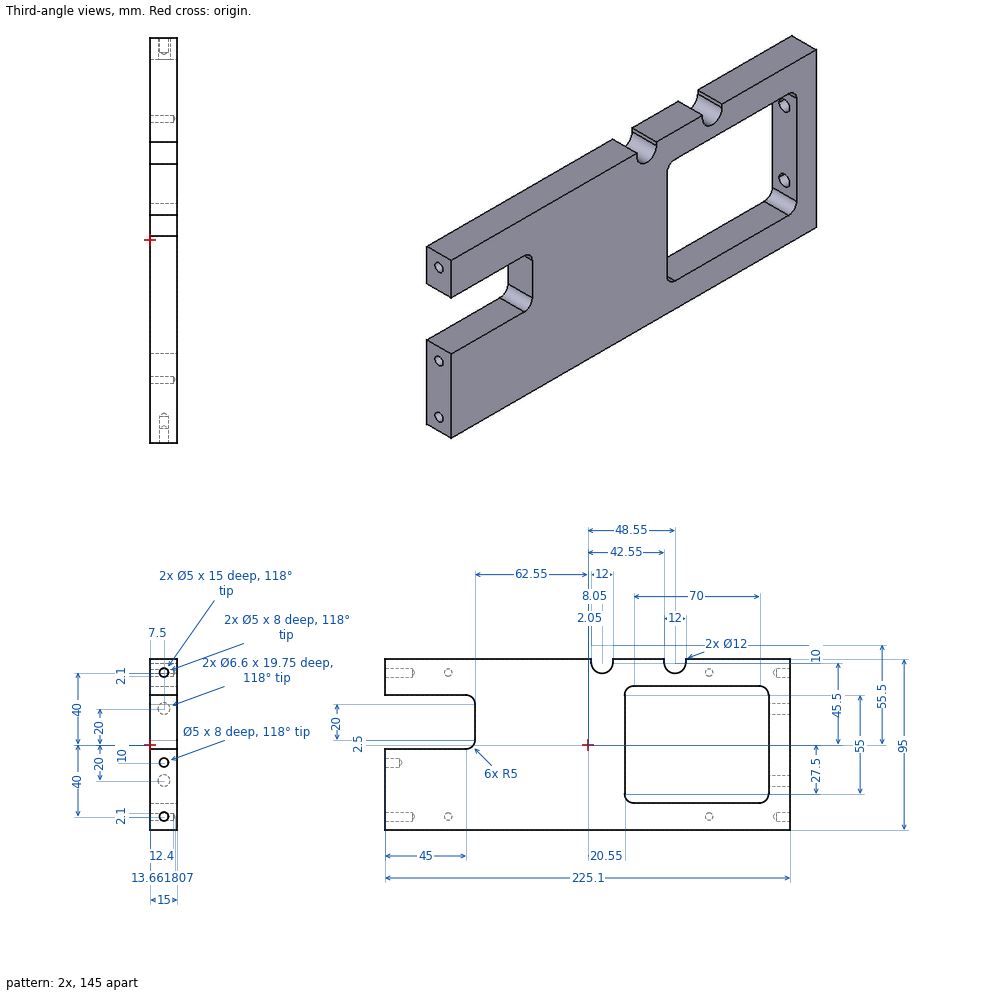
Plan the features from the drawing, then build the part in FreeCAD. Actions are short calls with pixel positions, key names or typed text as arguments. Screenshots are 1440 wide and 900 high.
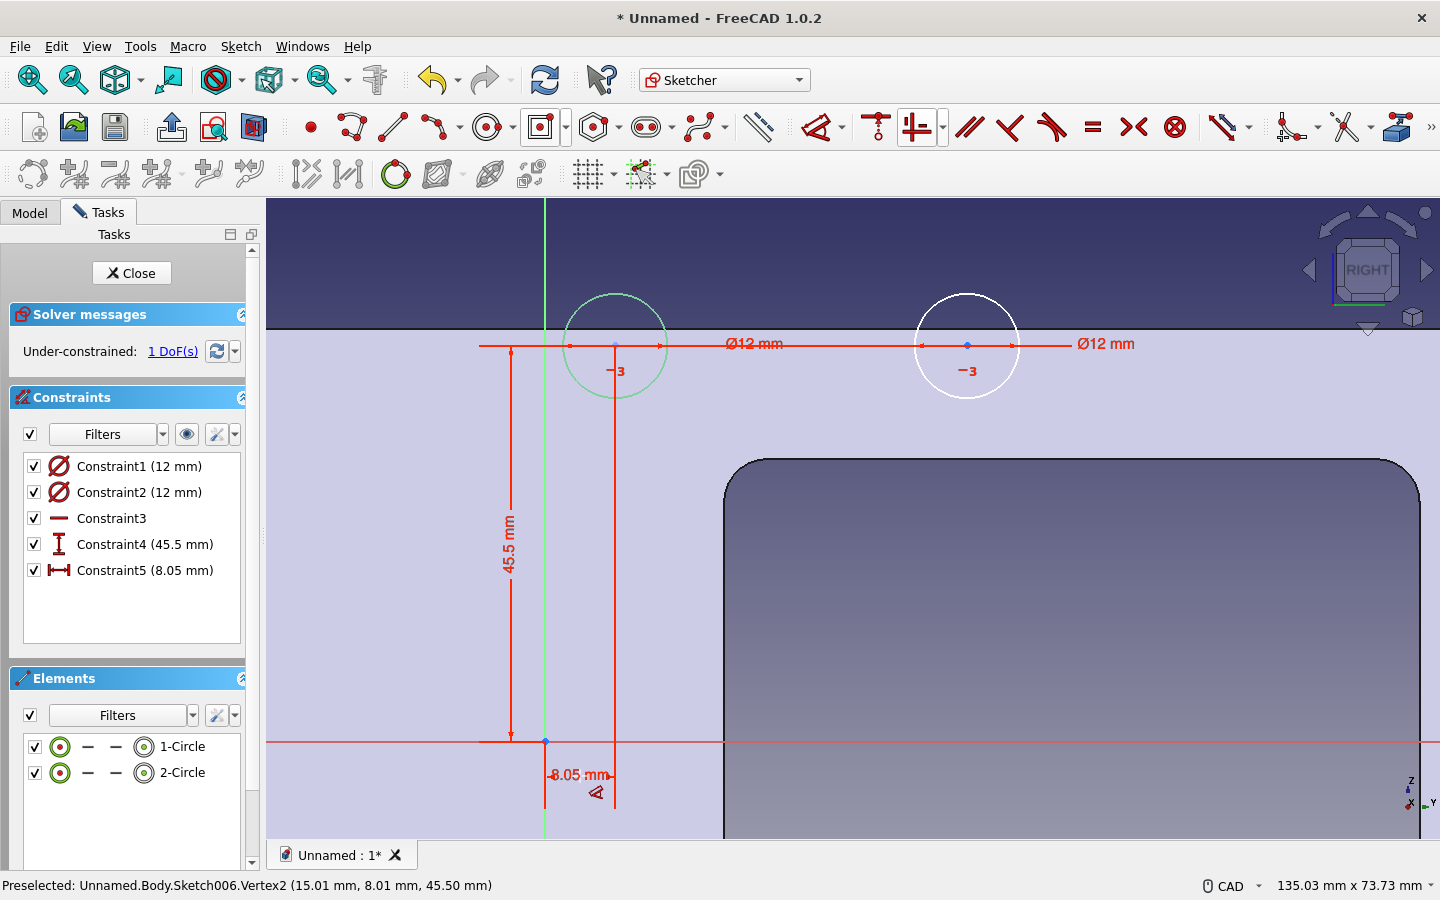
click(967, 346)
click(756, 776)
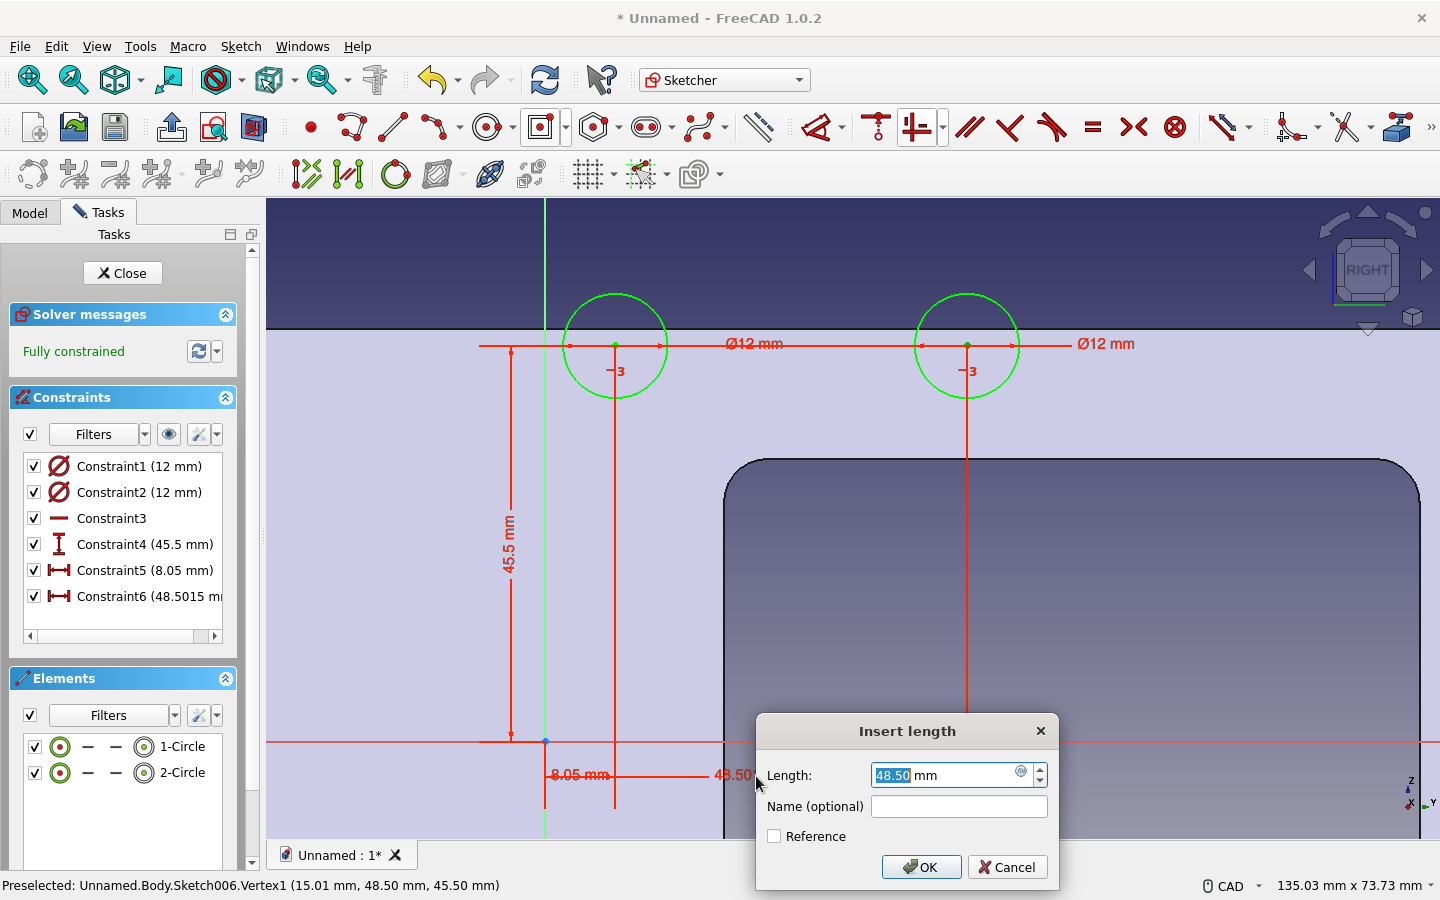
text(48.55)
key(Return)
key(Escape)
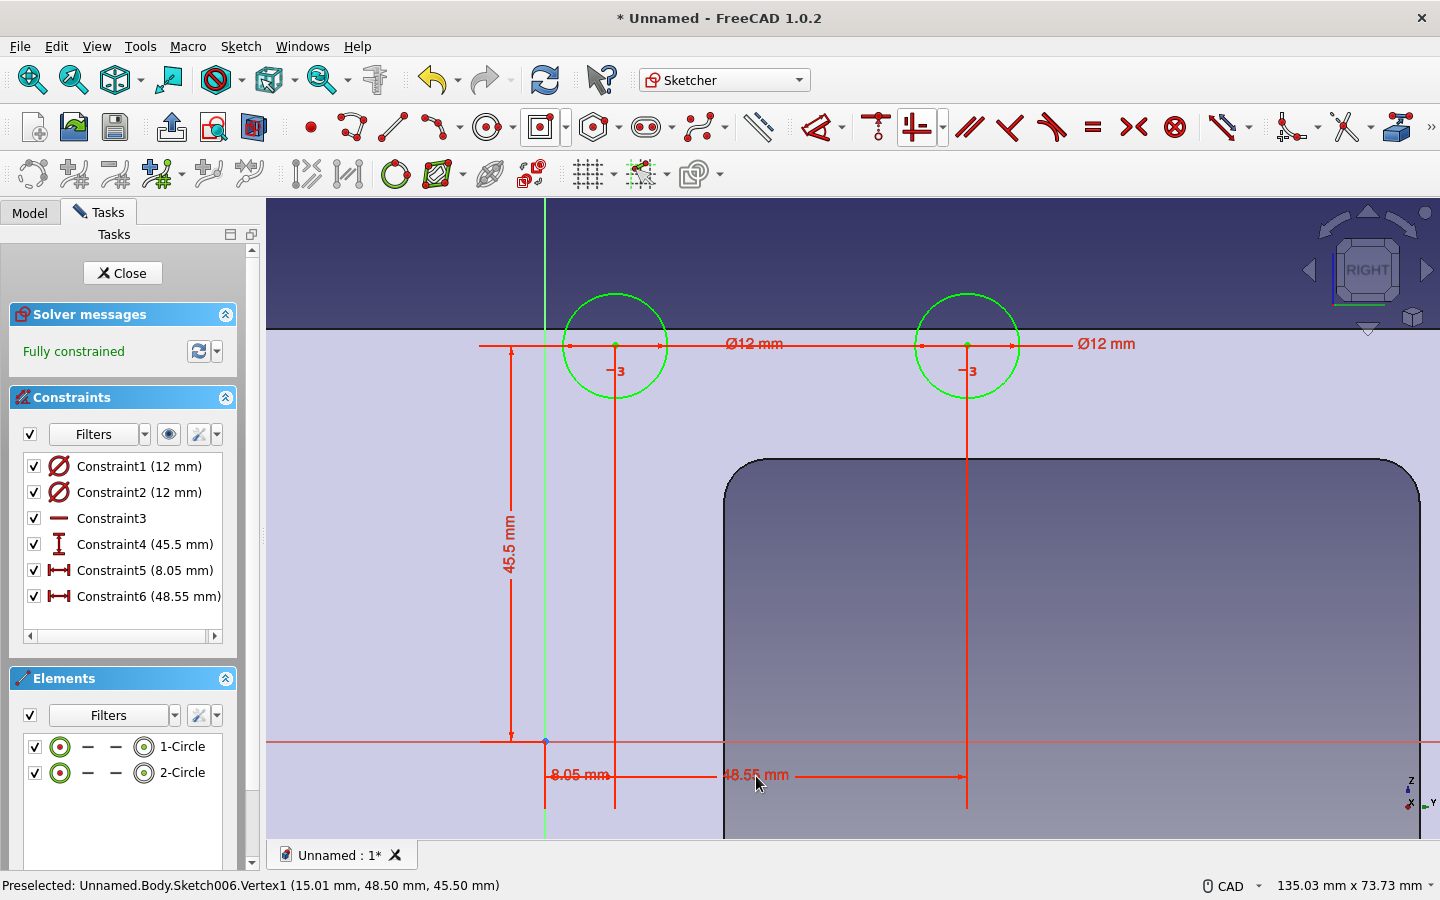
click(123, 273)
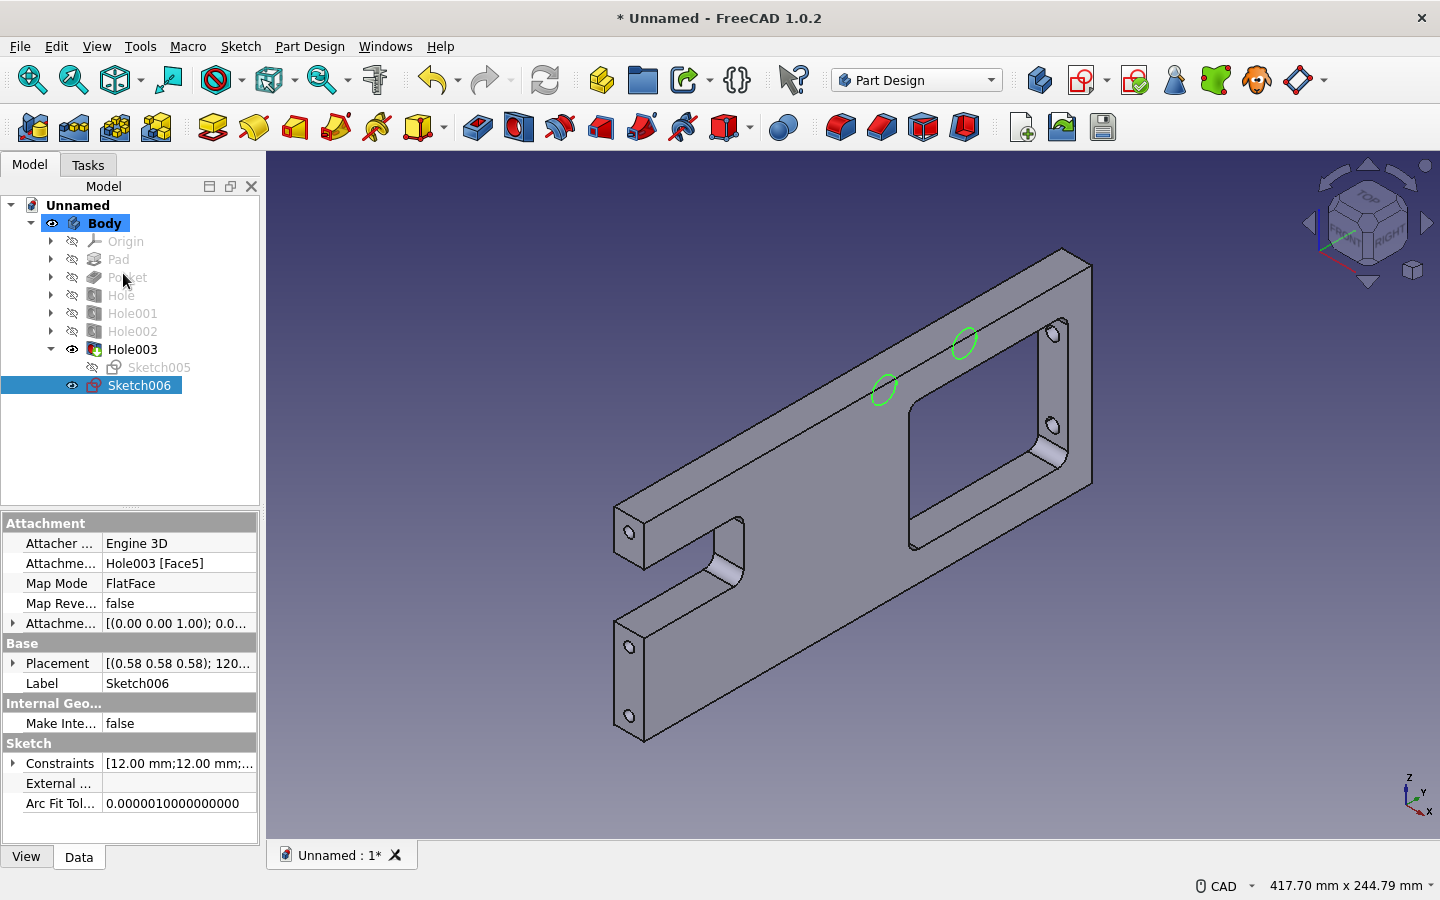
click(478, 128)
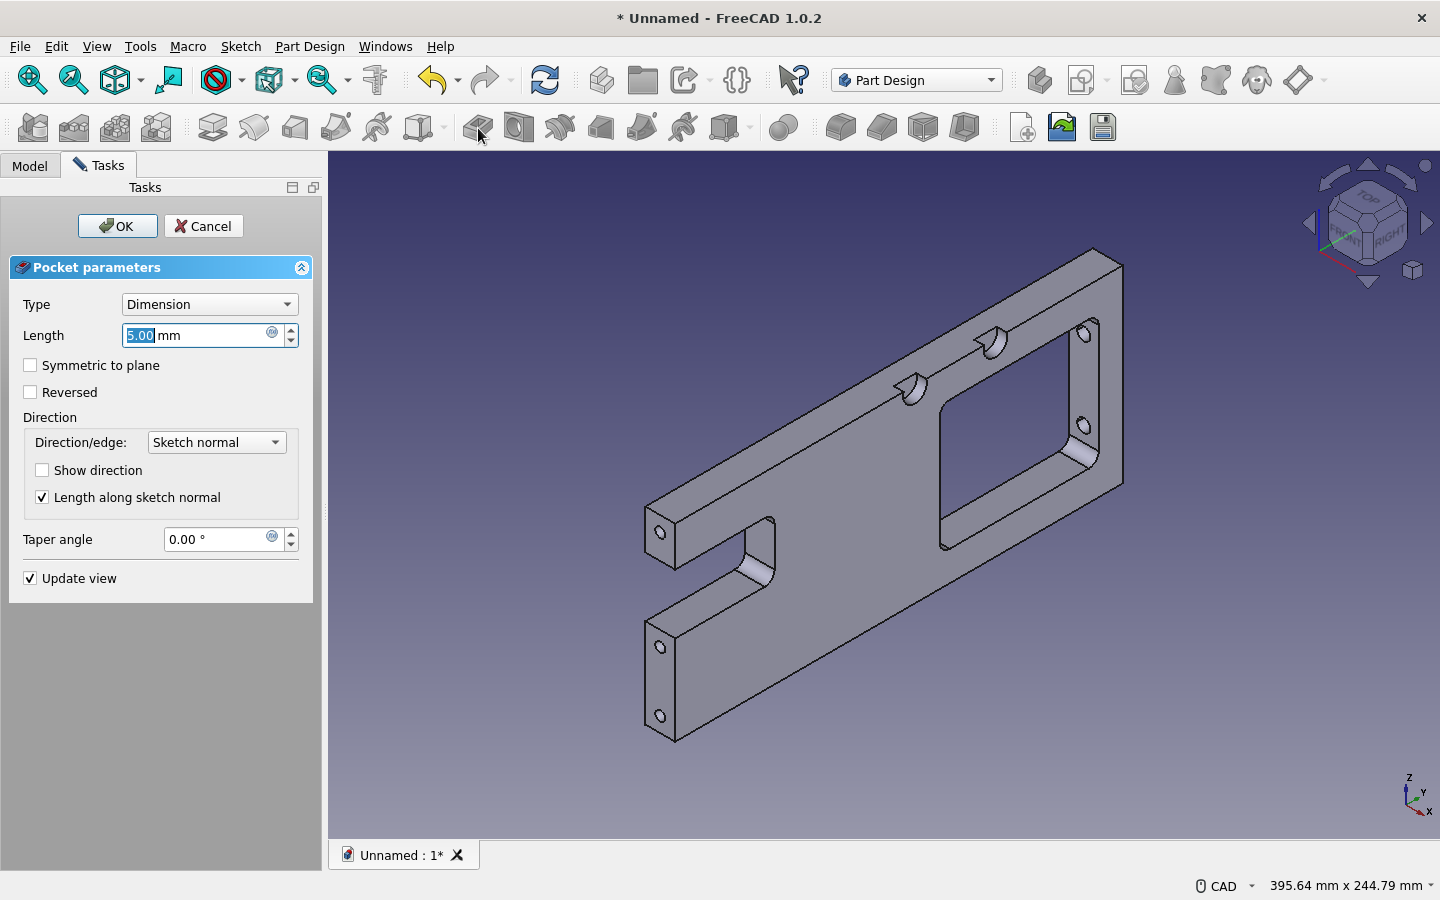
click(210, 304)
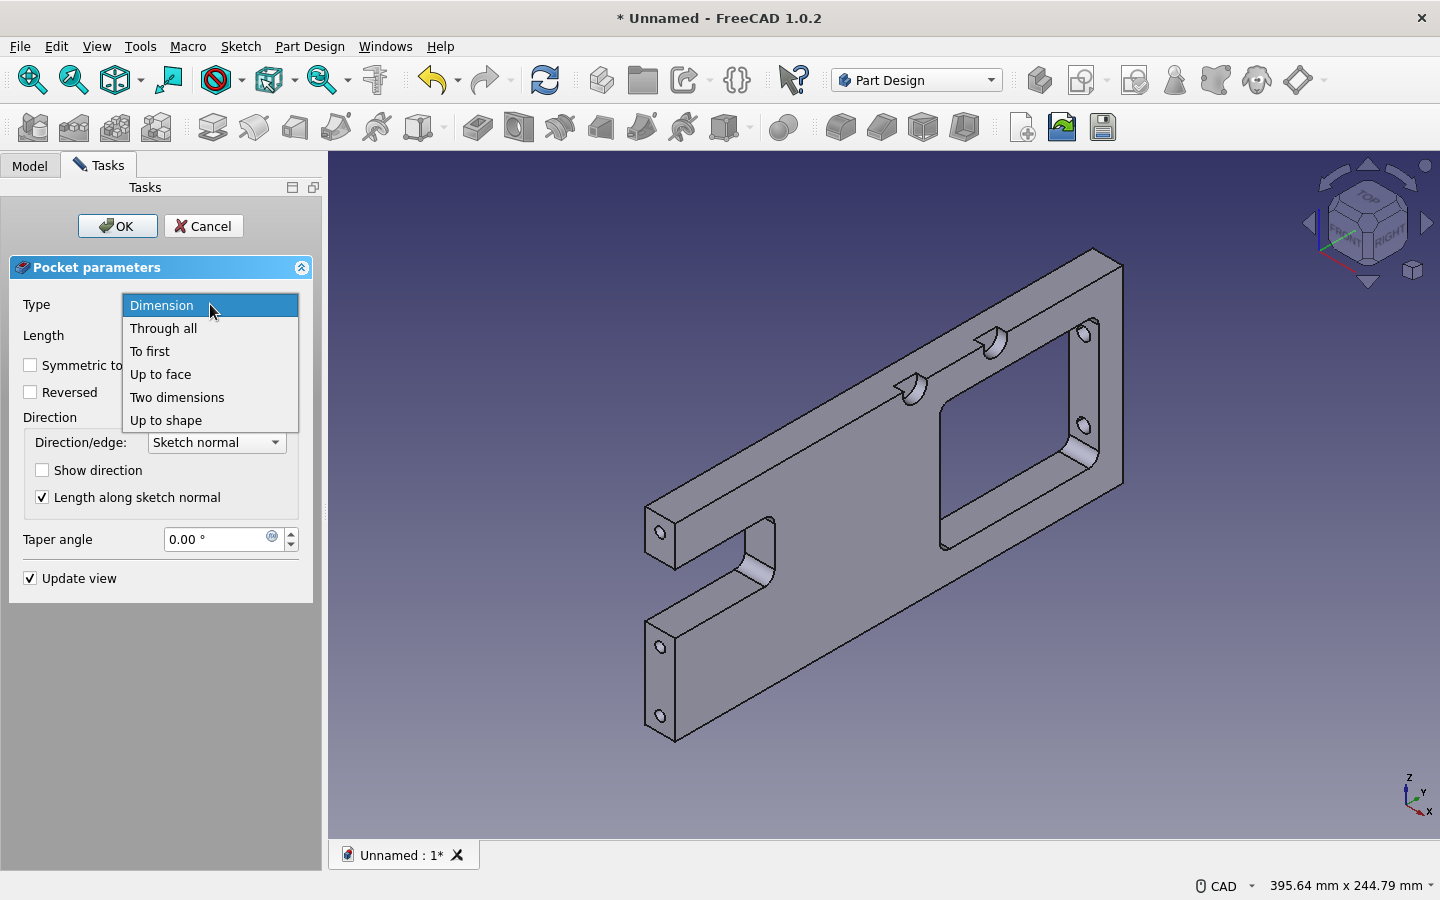
click(208, 328)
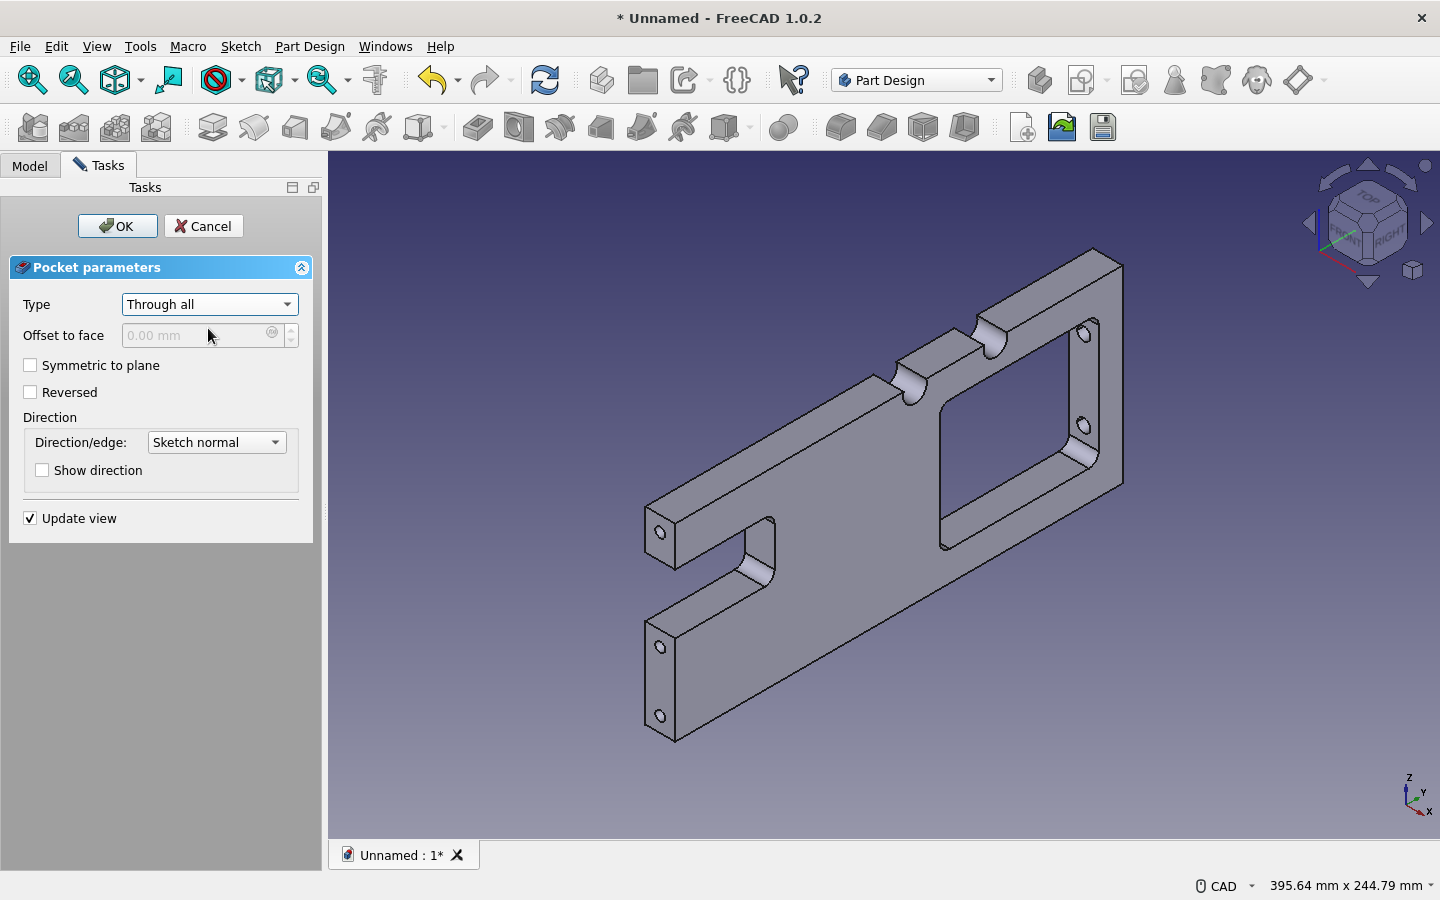
click(118, 226)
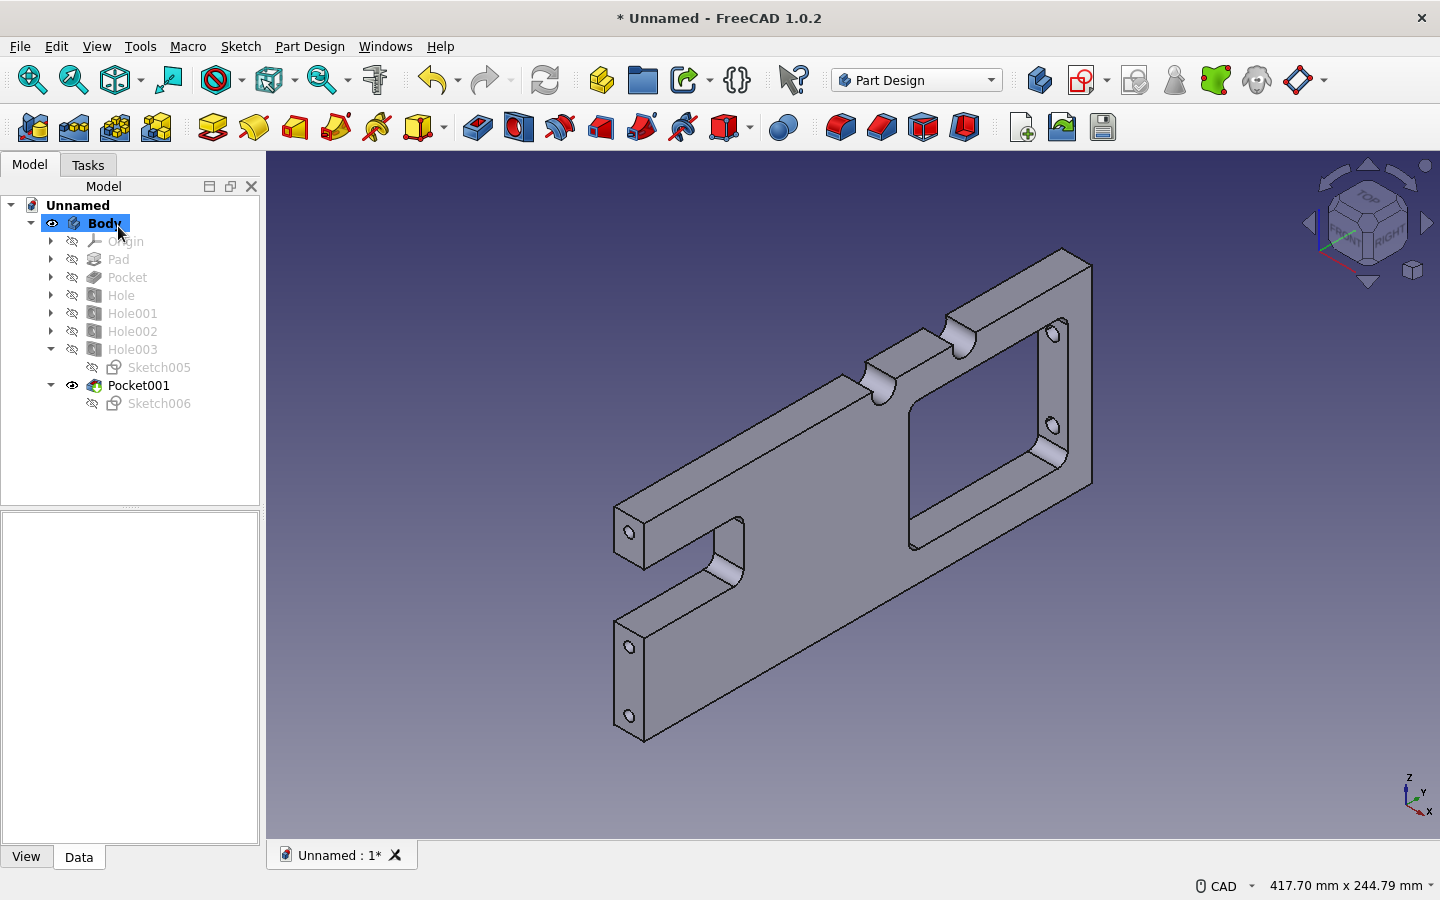
click(1080, 80)